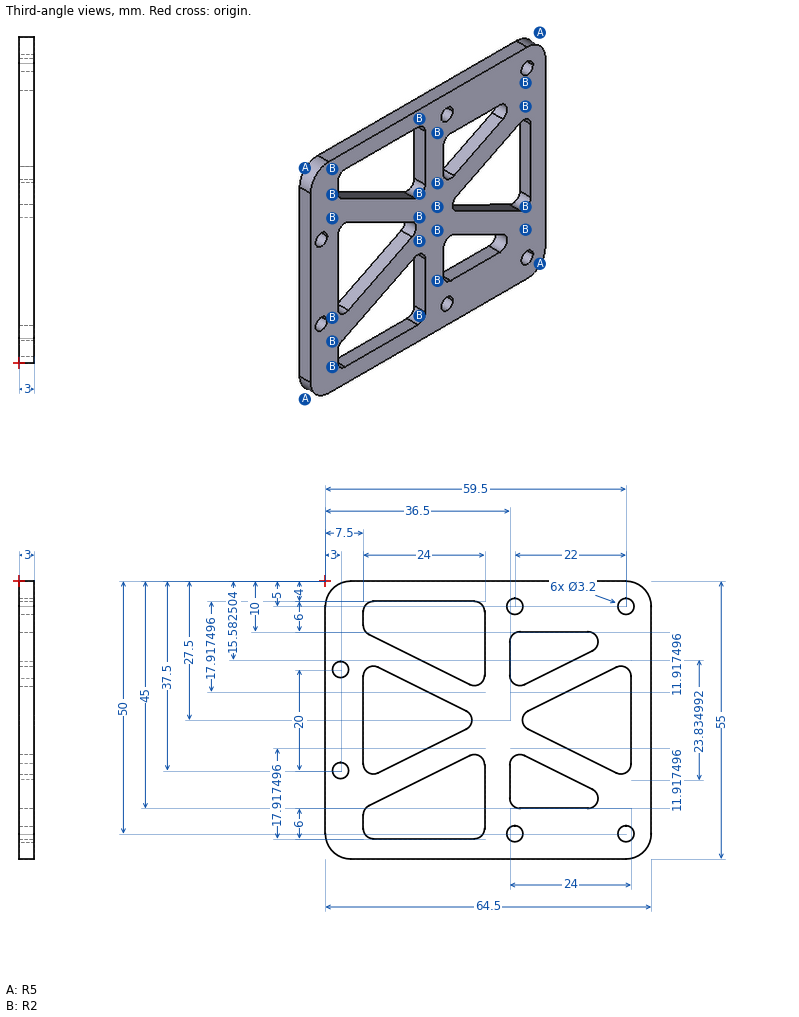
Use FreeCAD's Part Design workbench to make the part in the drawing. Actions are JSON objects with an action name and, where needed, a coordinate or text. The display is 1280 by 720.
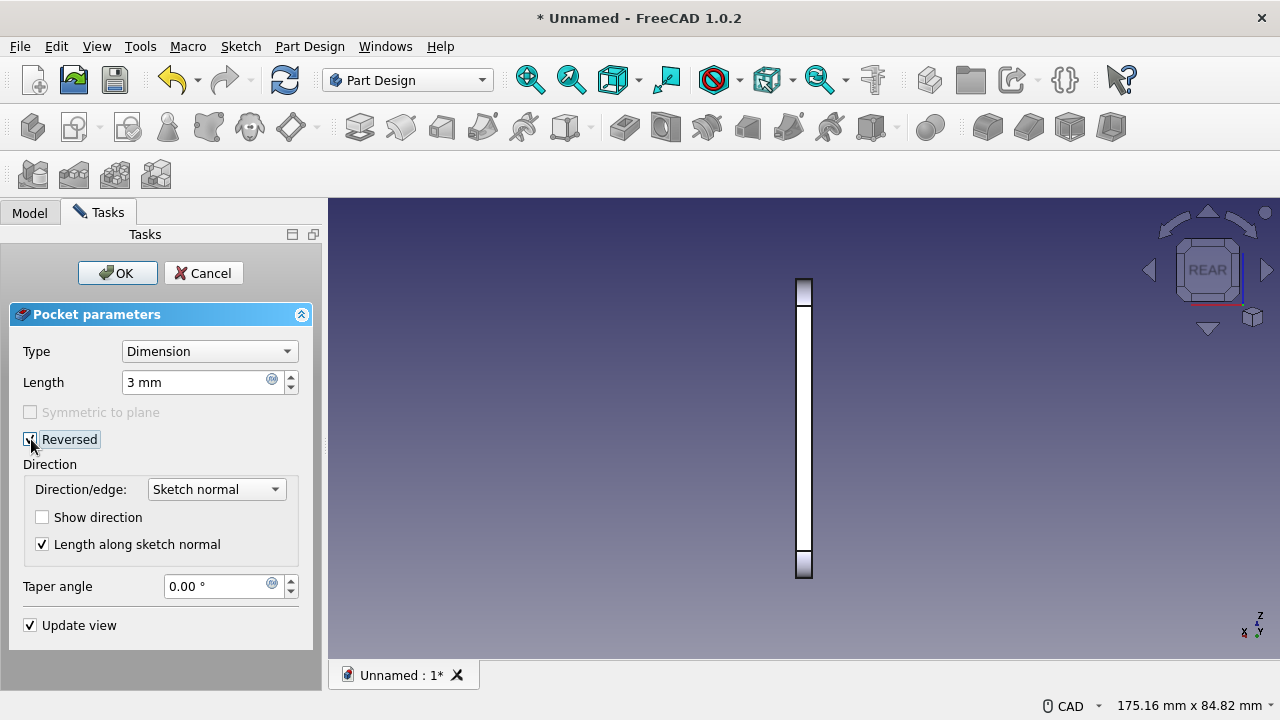
{"action": "left_click", "coordinate": [118, 273]}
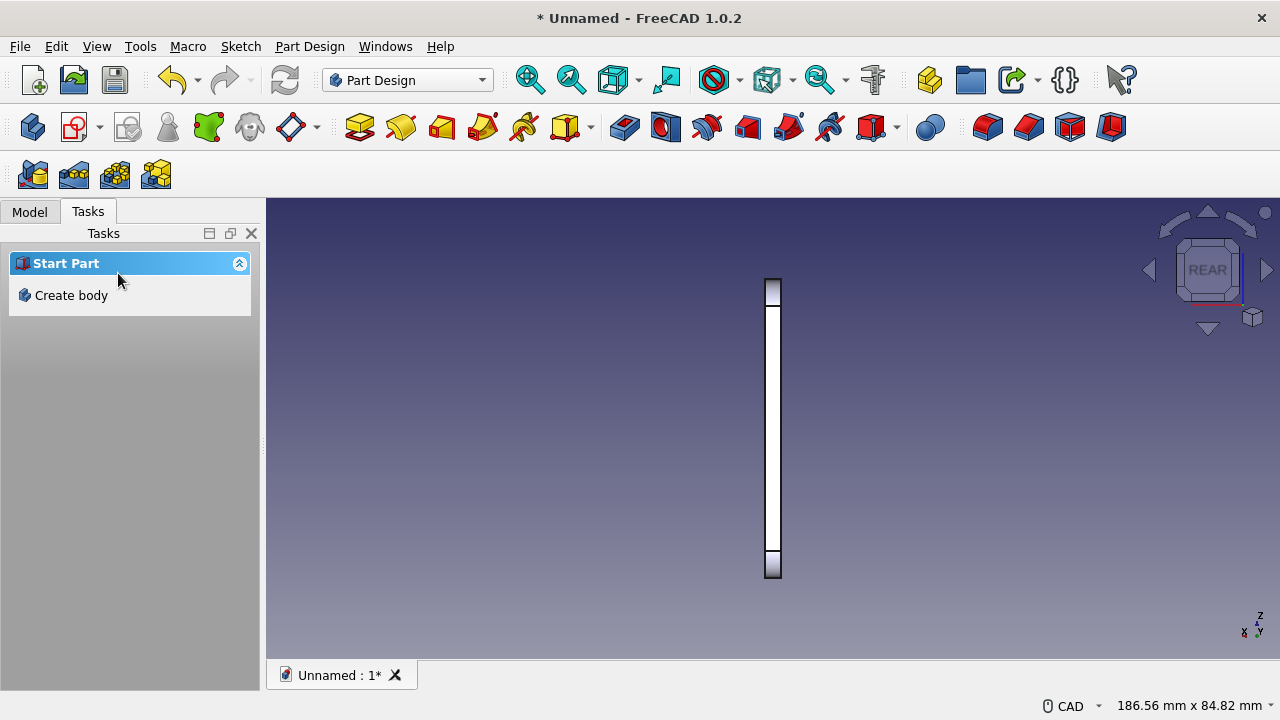
{"action": "scroll", "coordinate": [773, 523], "scroll_direction": "up", "scroll_amount": 5}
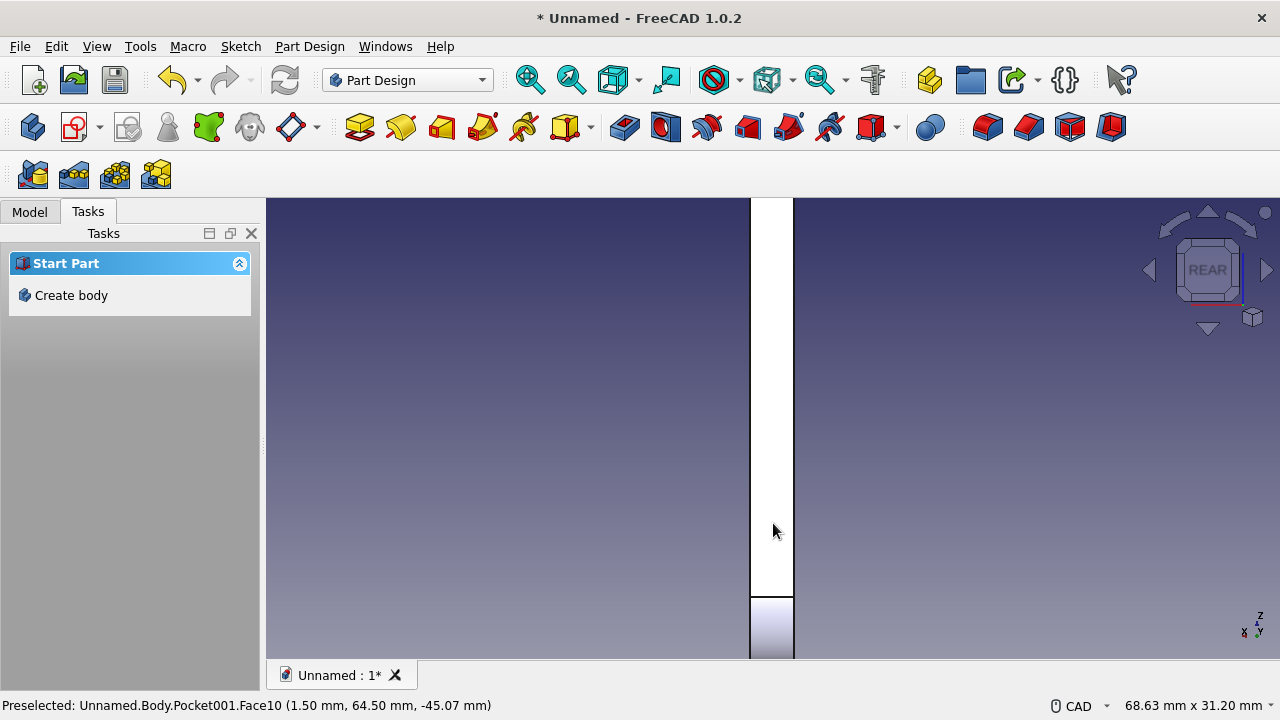
{"action": "left_click", "coordinate": [531, 80]}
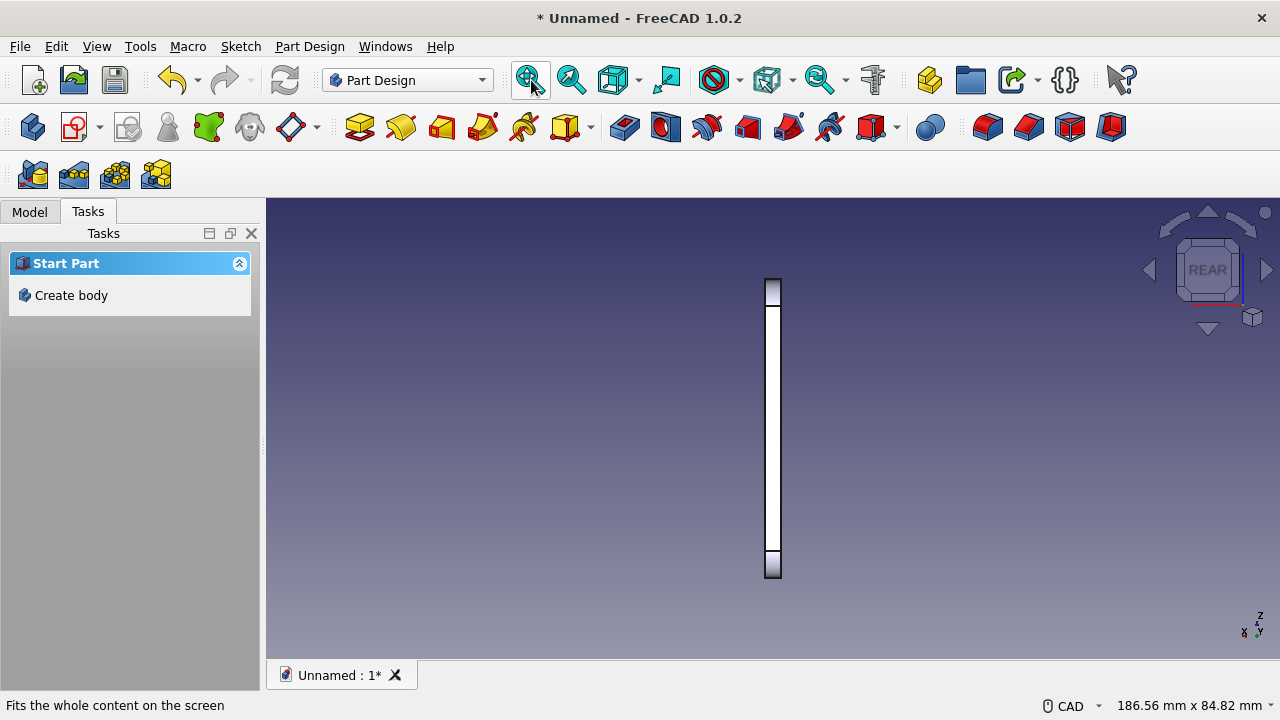
{"action": "key", "text": "0"}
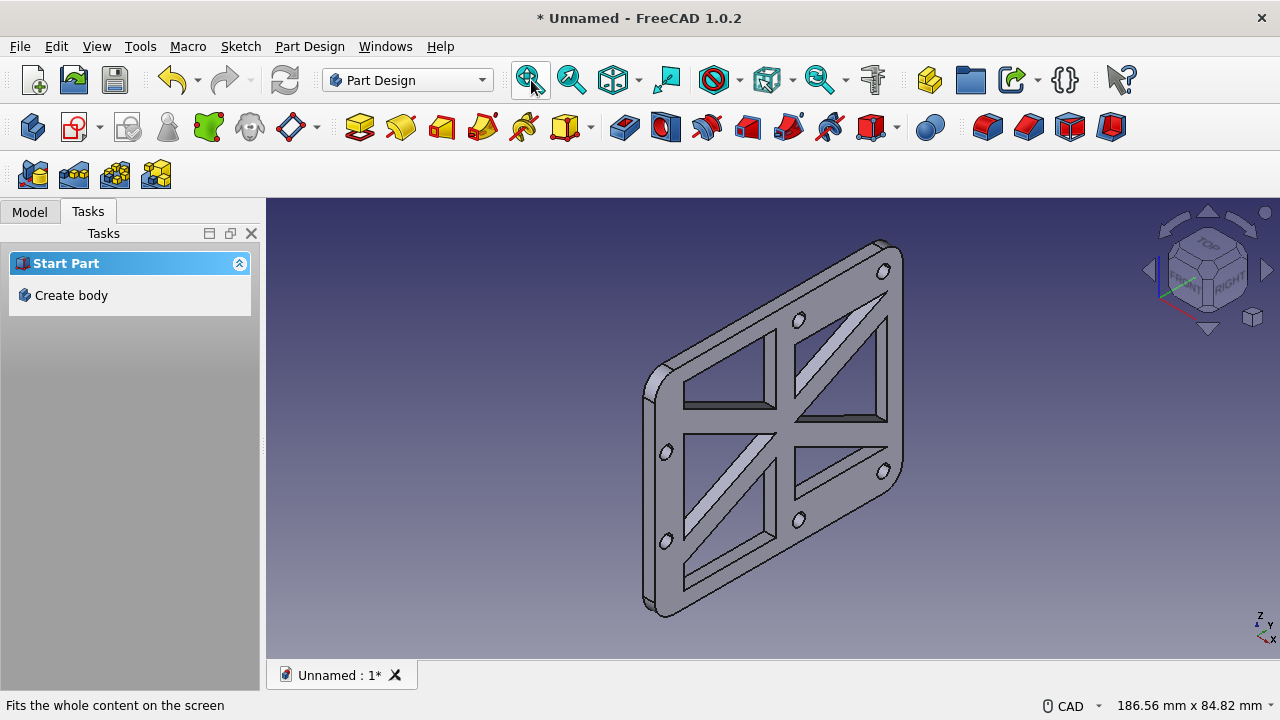
{"action": "scroll", "coordinate": [882, 442], "scroll_direction": "up", "scroll_amount": 5}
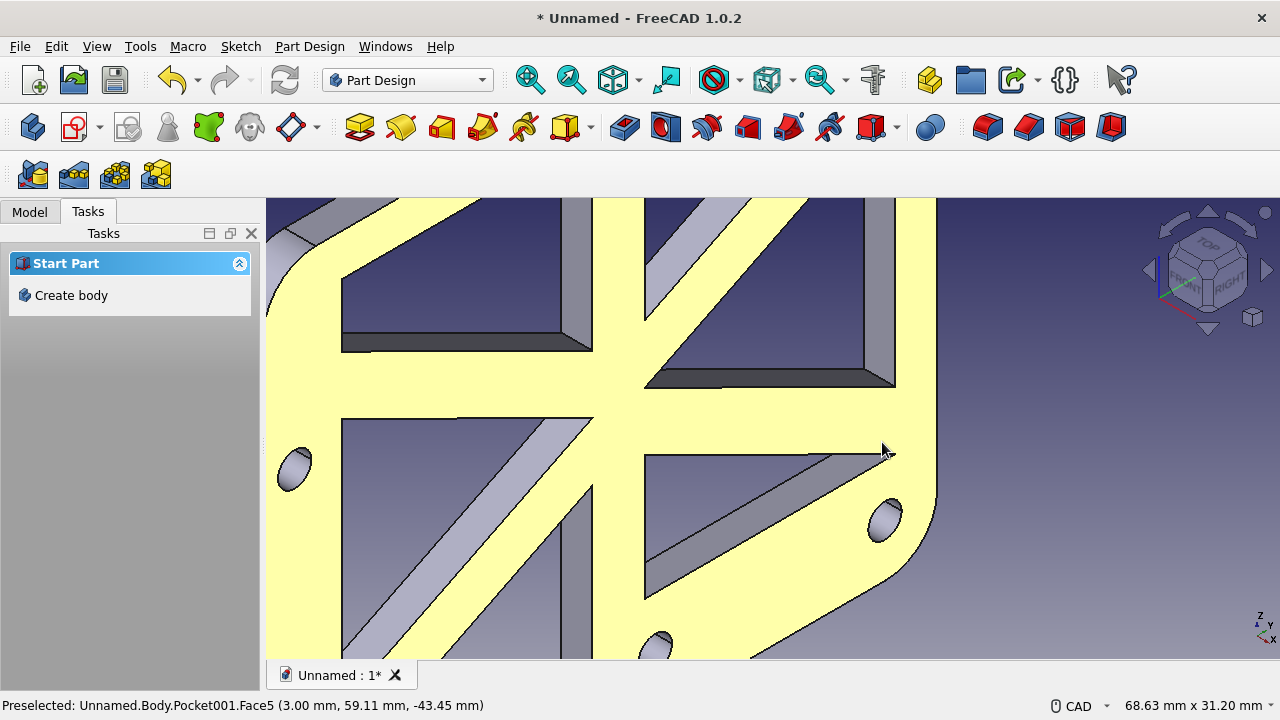
{"action": "left_click", "coordinate": [531, 80]}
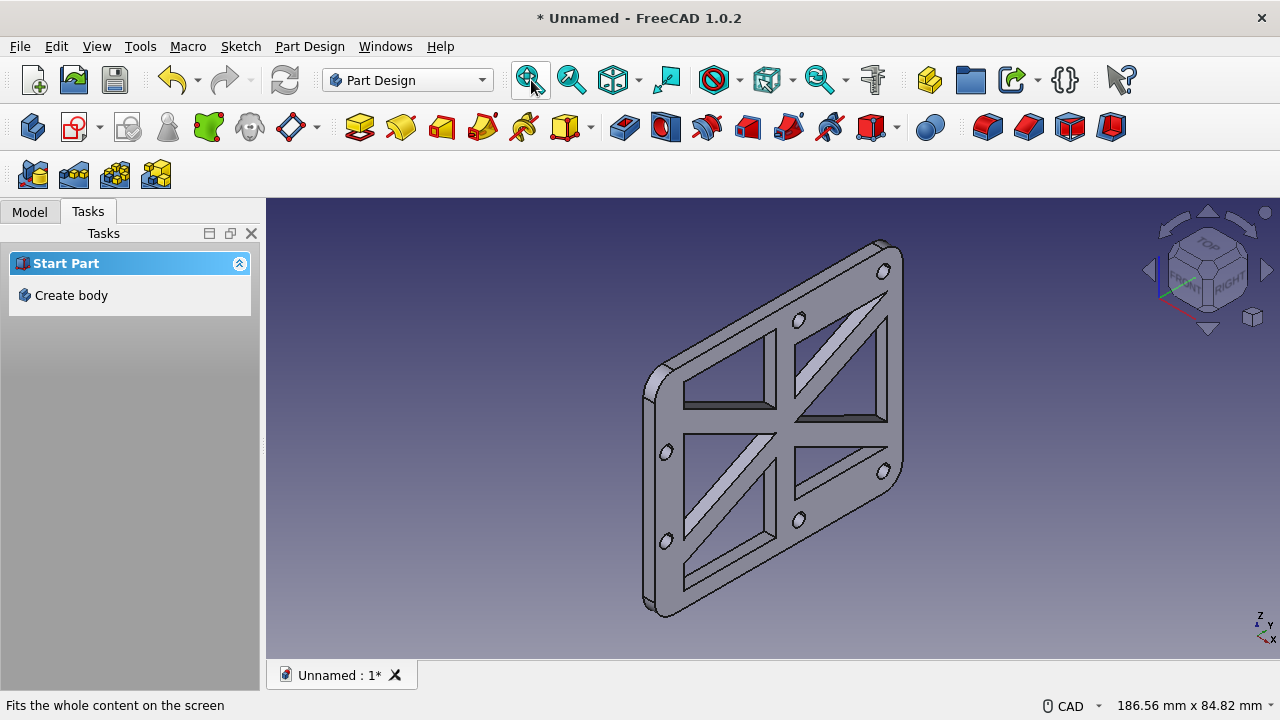
{"action": "key", "text": "2"}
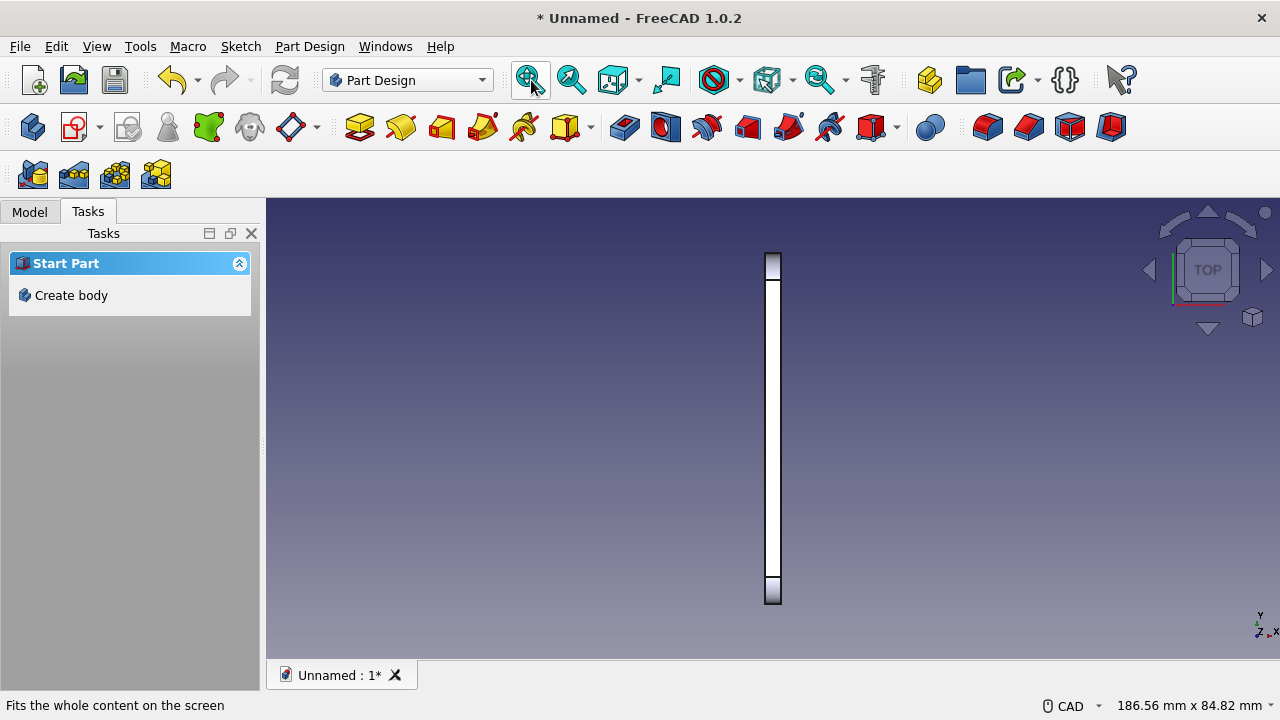
{"action": "scroll", "coordinate": [773, 274], "scroll_direction": "up", "scroll_amount": 5}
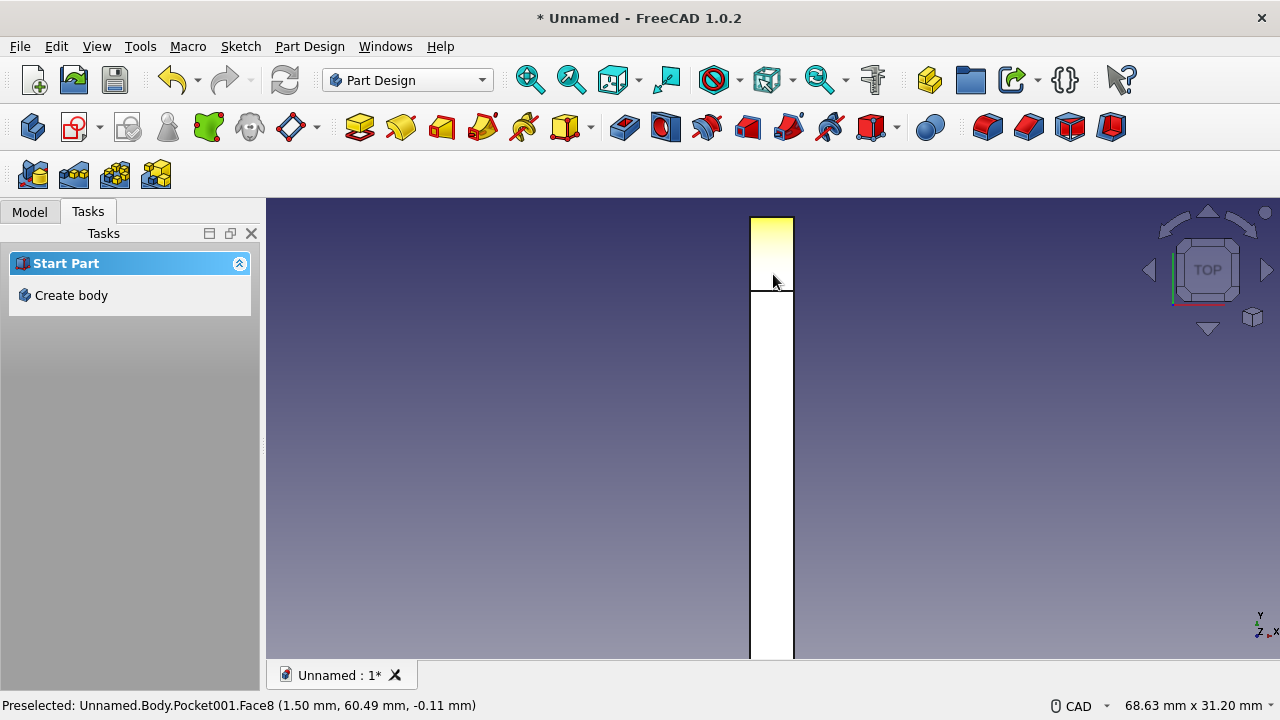
{"action": "left_click", "coordinate": [531, 80]}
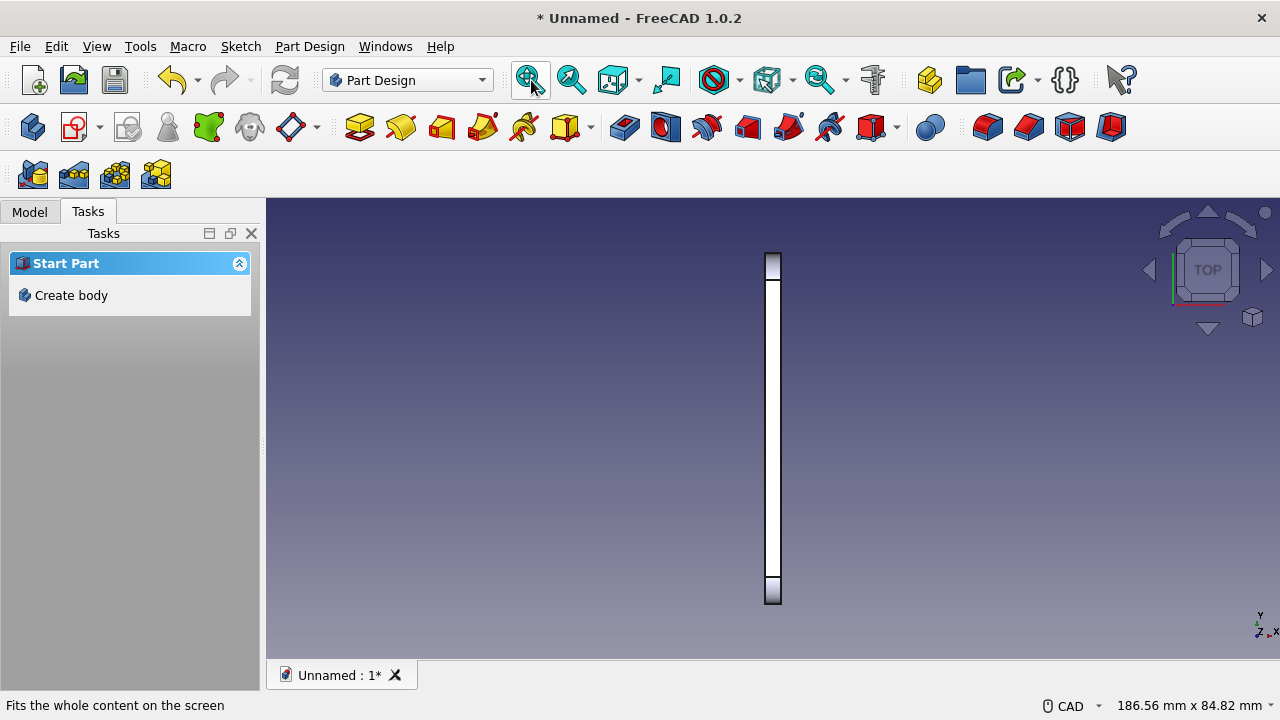
{"action": "key", "text": "1"}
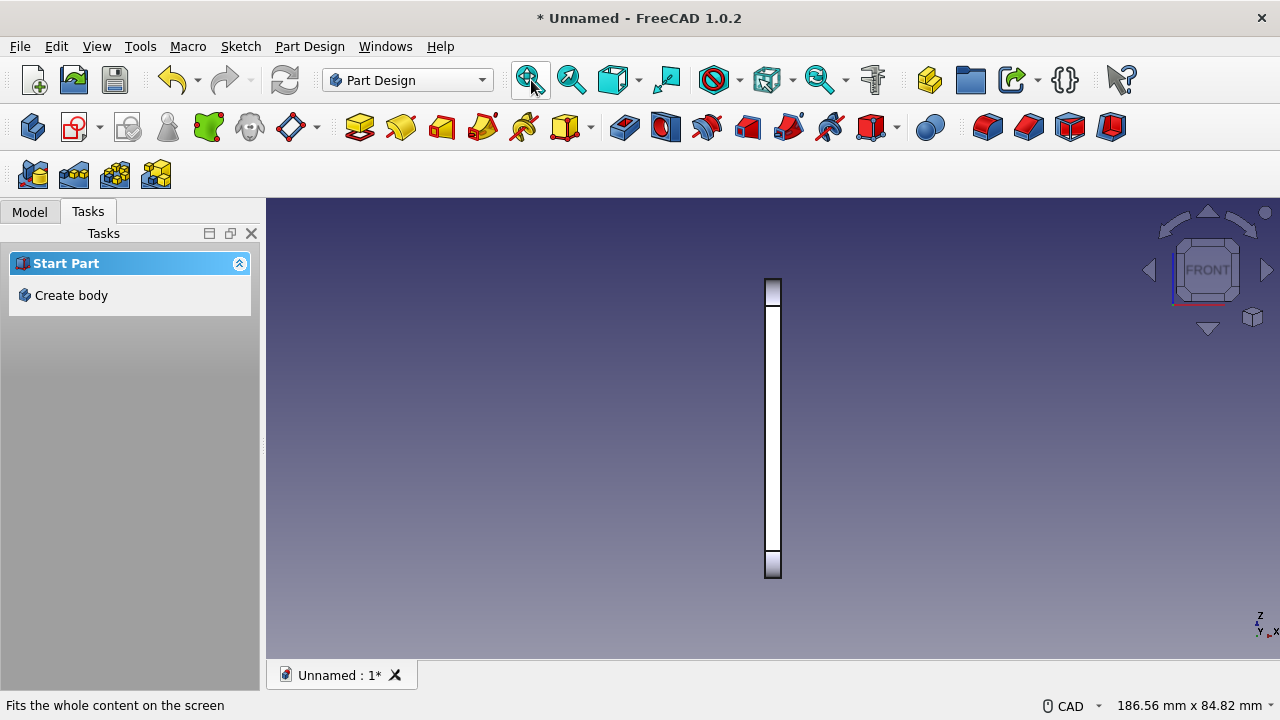
{"action": "scroll", "coordinate": [773, 523], "scroll_direction": "up", "scroll_amount": 5}